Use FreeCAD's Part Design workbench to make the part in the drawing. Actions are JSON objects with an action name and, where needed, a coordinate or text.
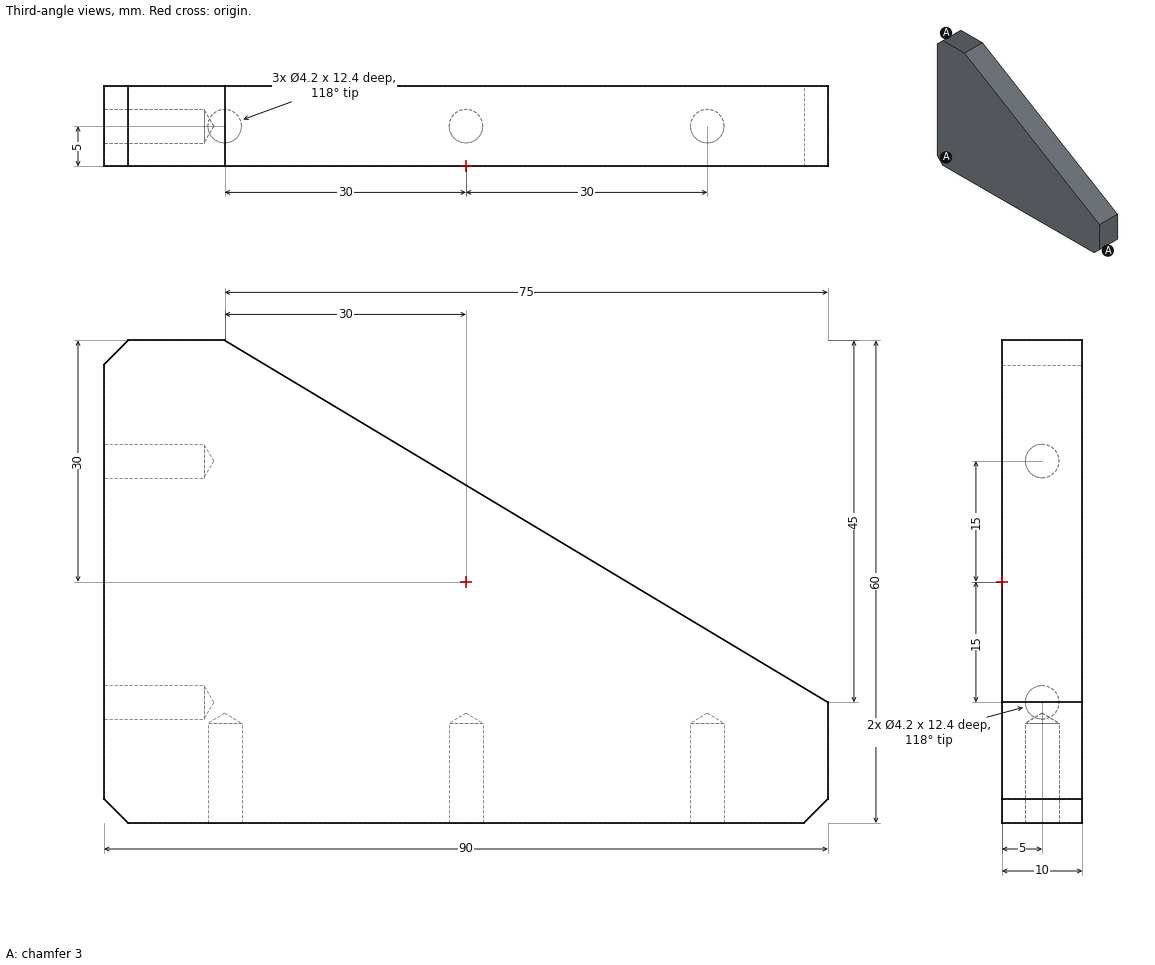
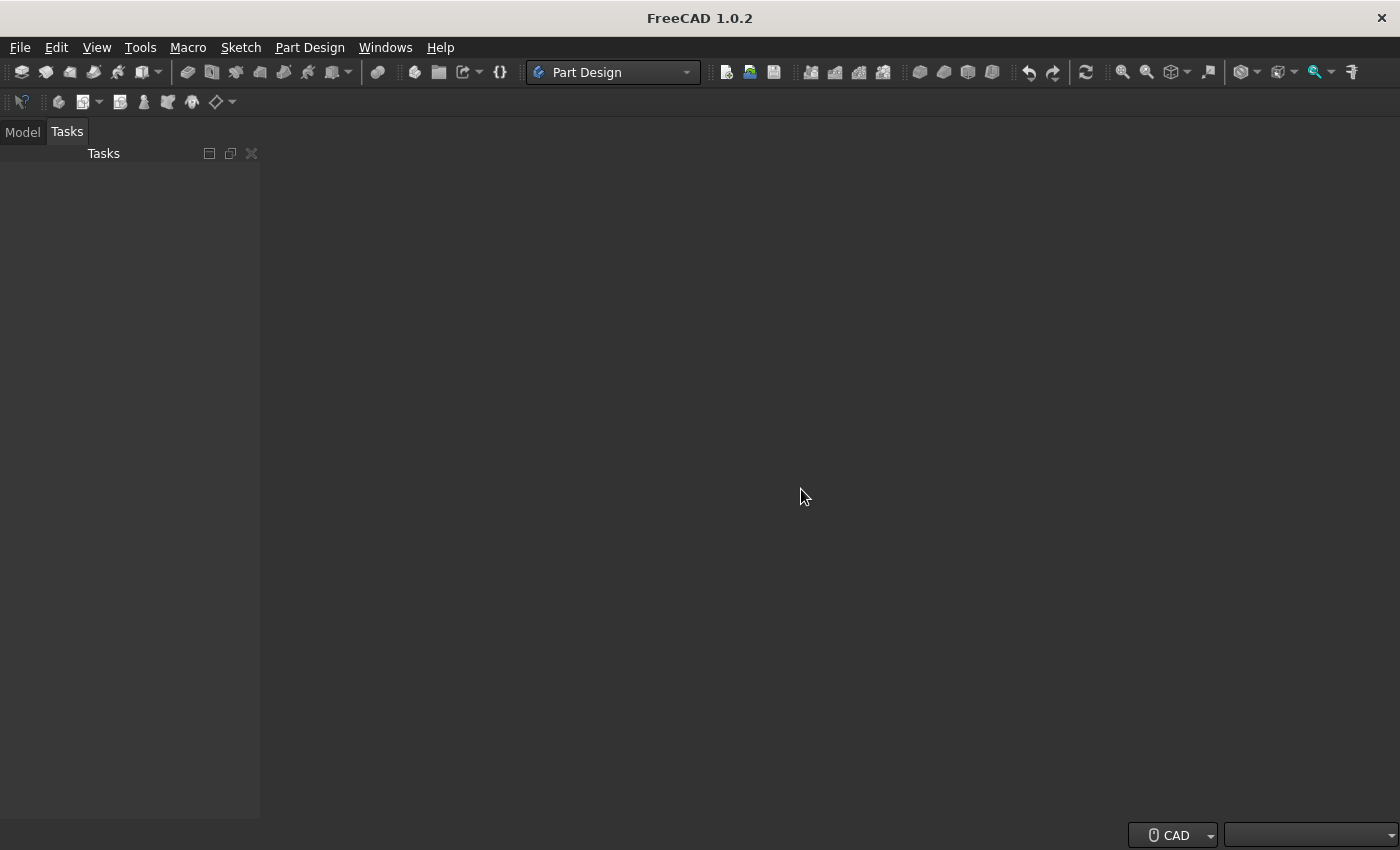
{"action": "key", "text": "ctrl+n"}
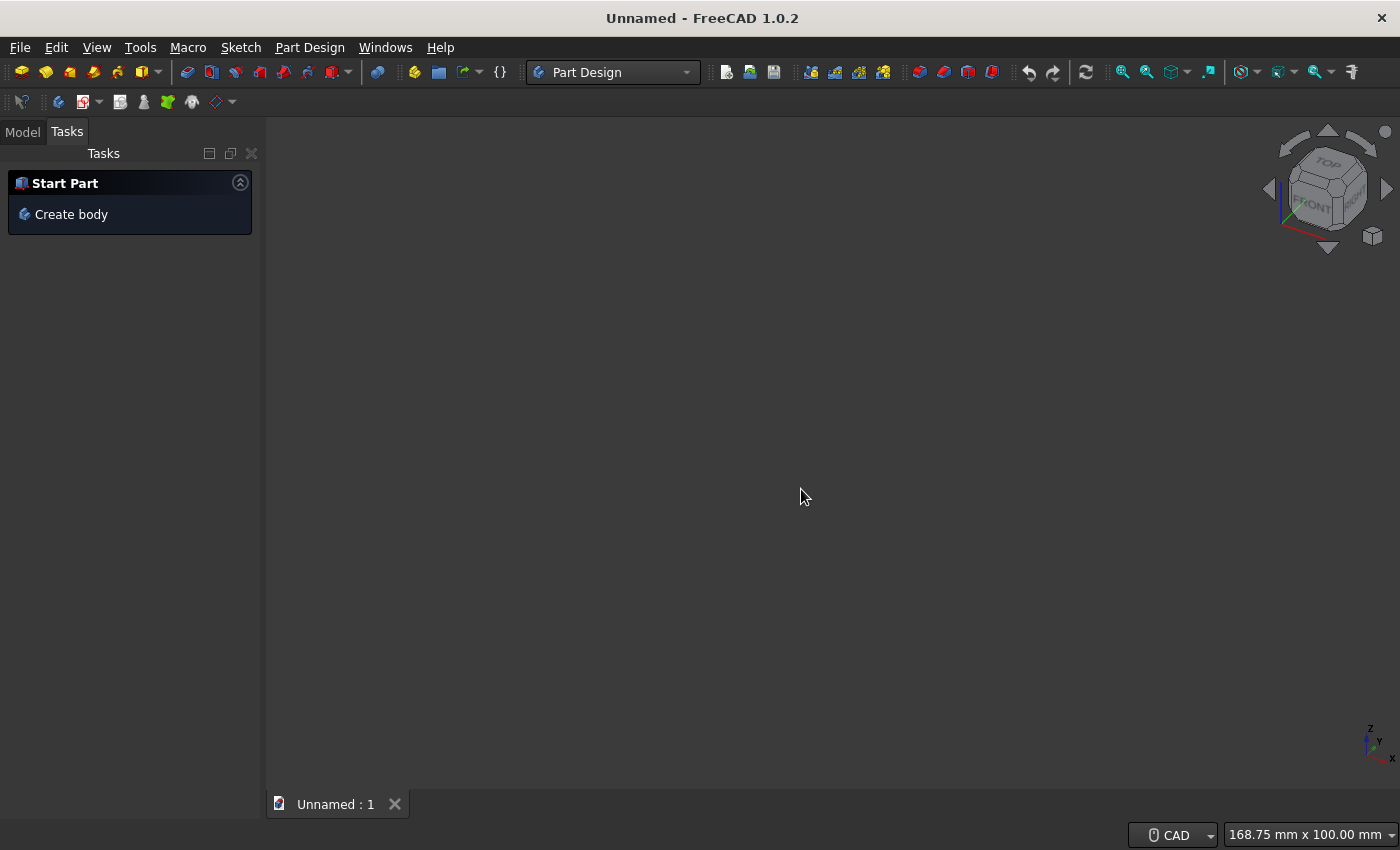
{"action": "left_click", "coordinate": [84, 102]}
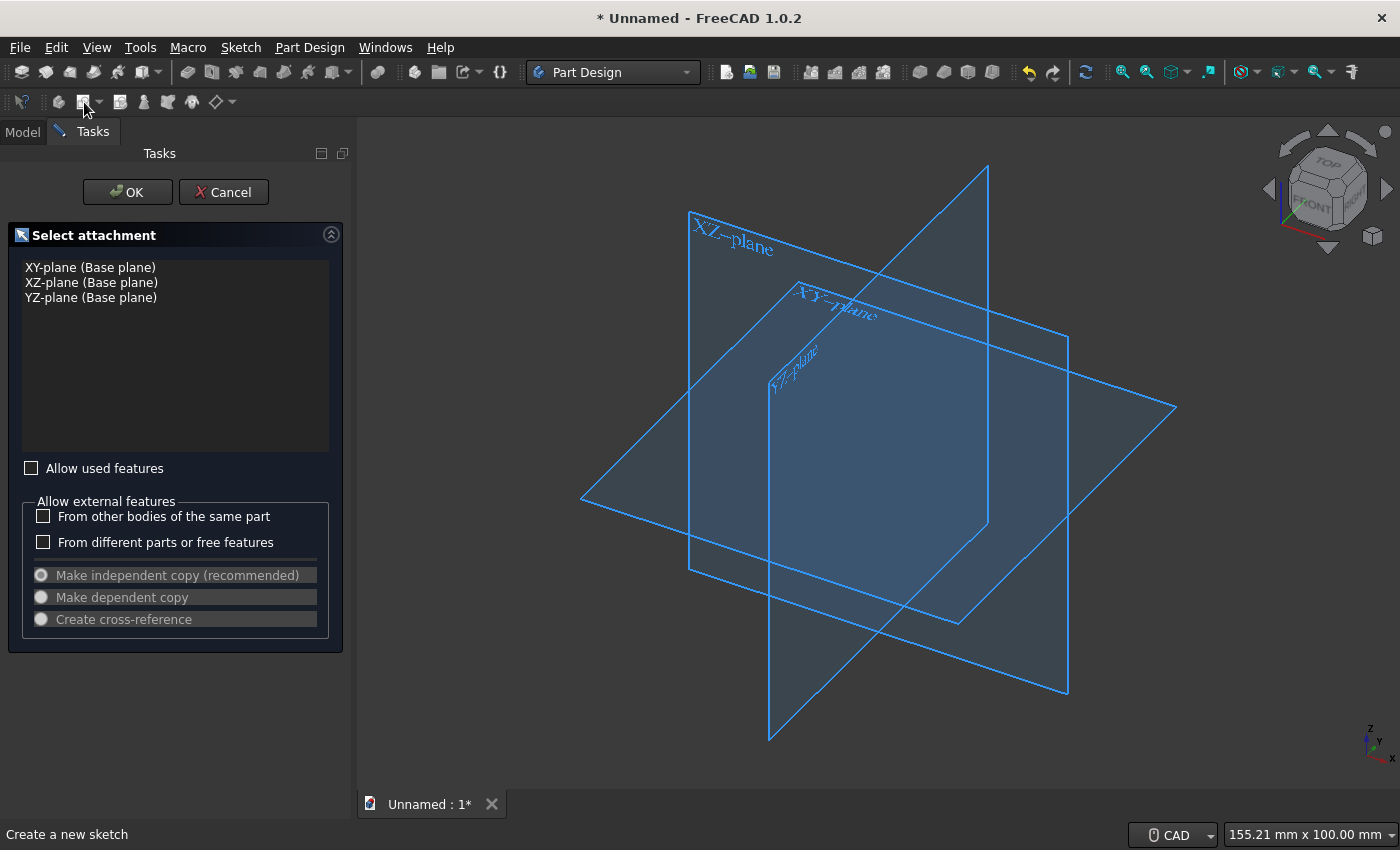
{"action": "left_click", "coordinate": [82, 282]}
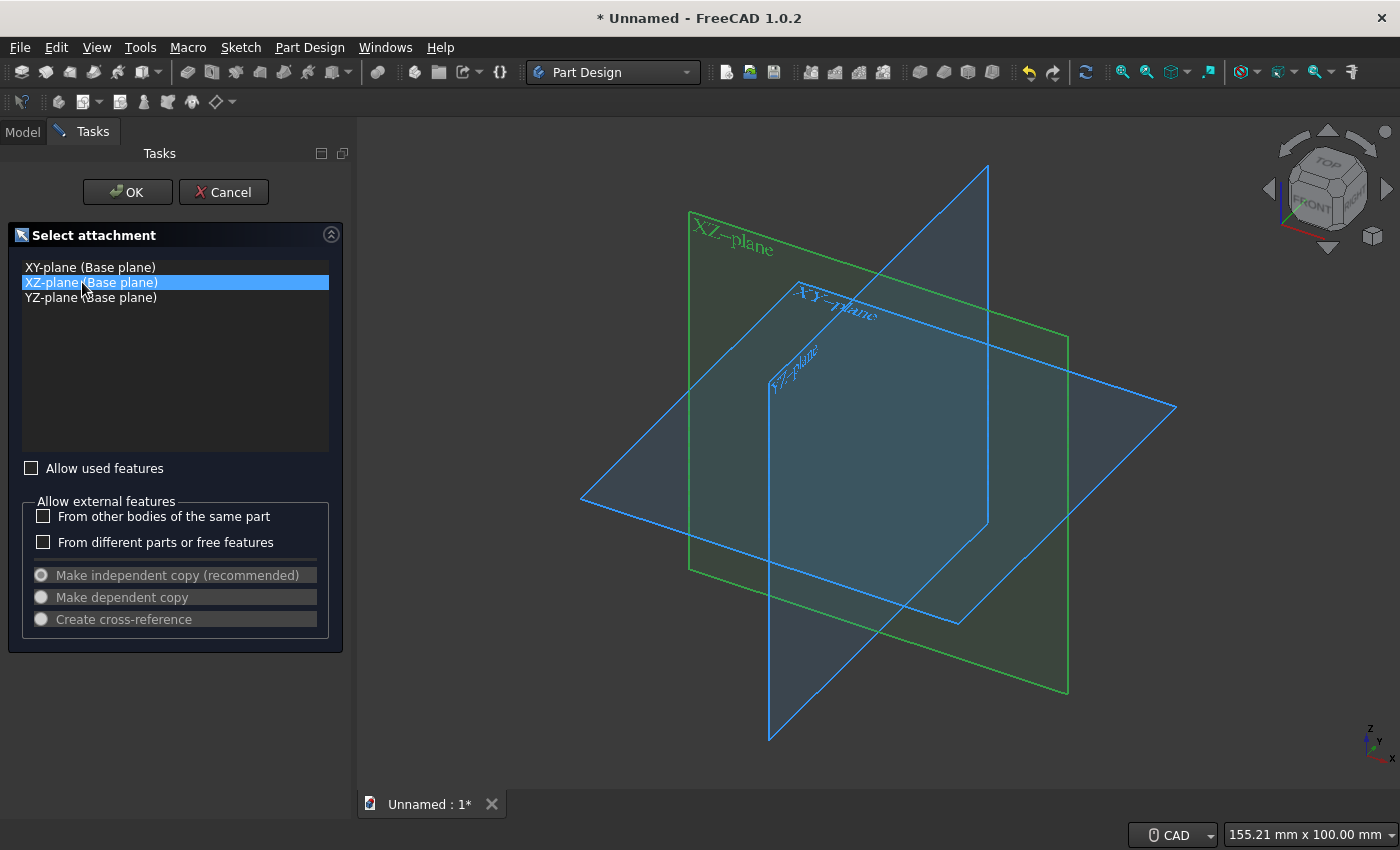
{"action": "left_click", "coordinate": [128, 192]}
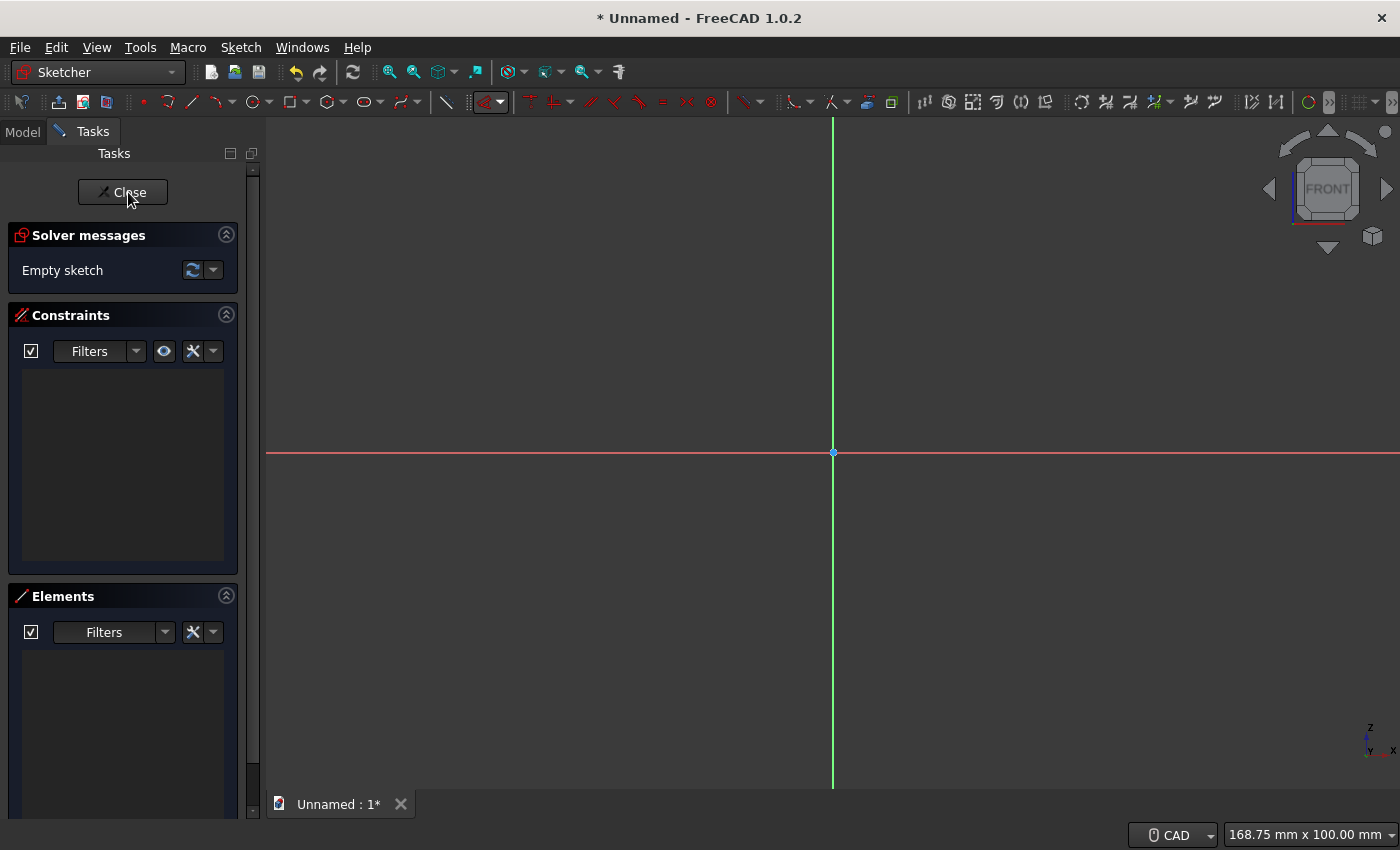
{"action": "key", "text": "g v"}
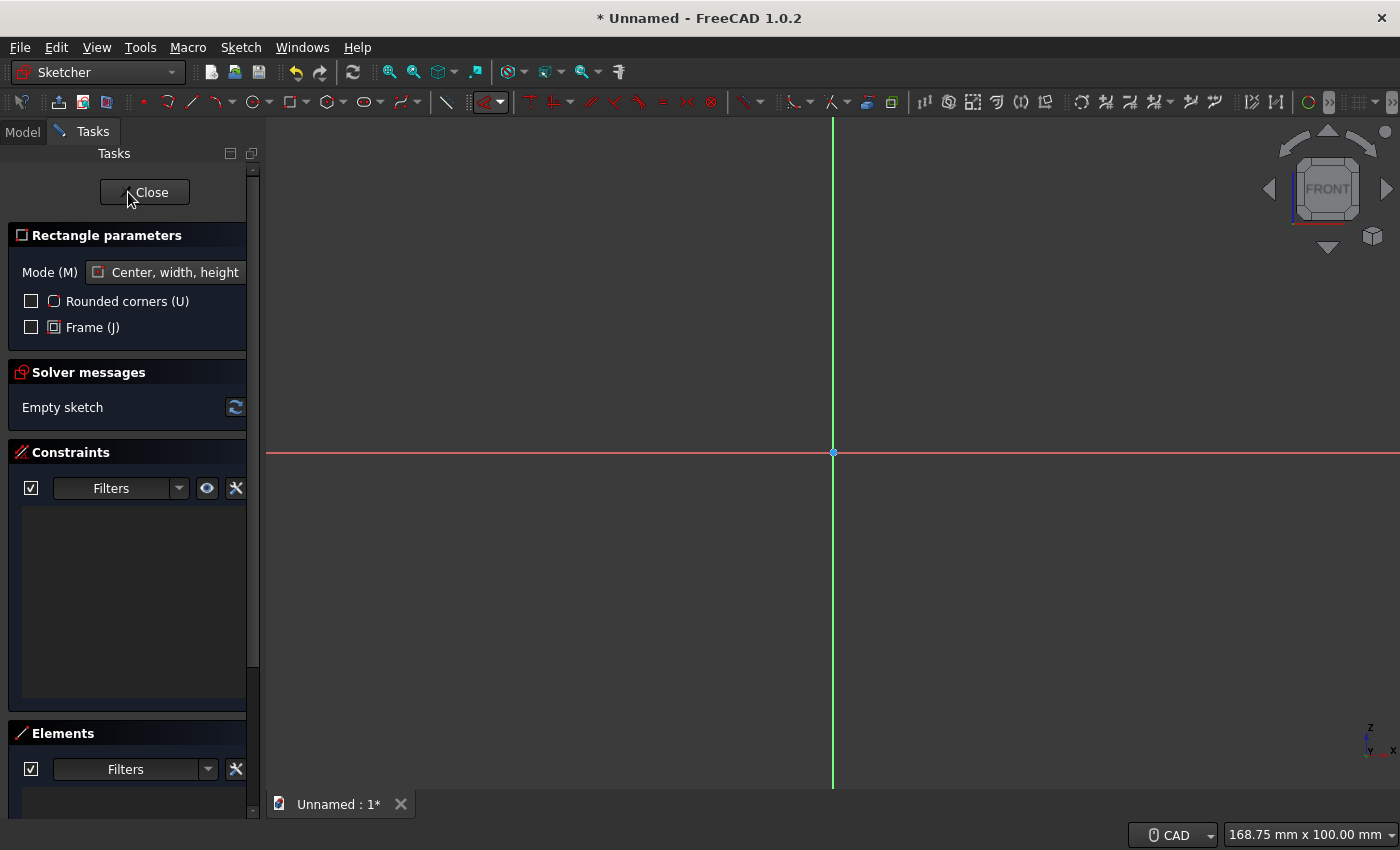
{"action": "left_click", "coordinate": [833, 453]}
{"action": "mouse_move", "coordinate": [1135, 251]}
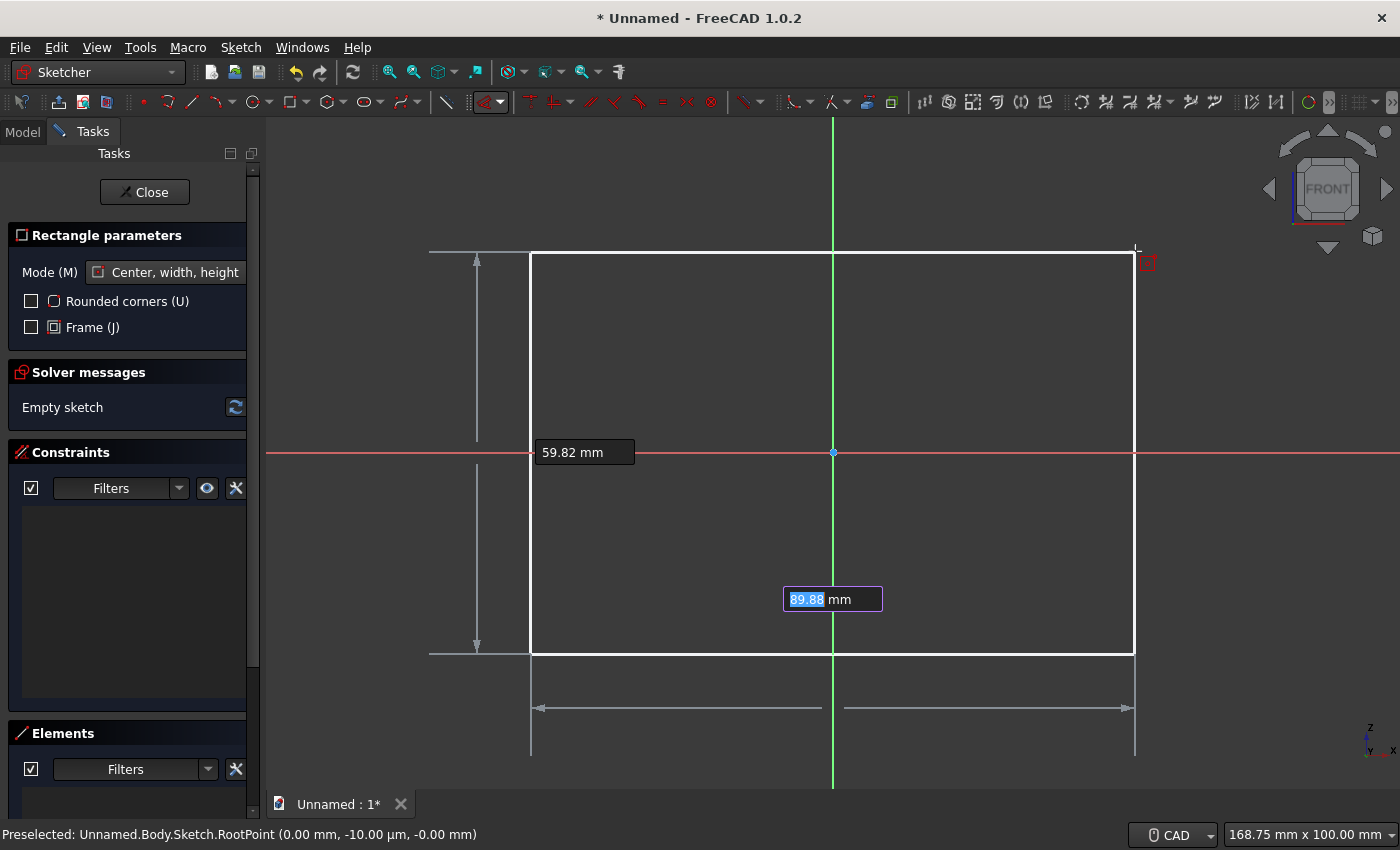
{"action": "type", "text": "90"}
{"action": "key", "text": "Tab"}
{"action": "type", "text": "60"}
{"action": "key", "text": "Return"}
{"action": "key", "text": "Escape"}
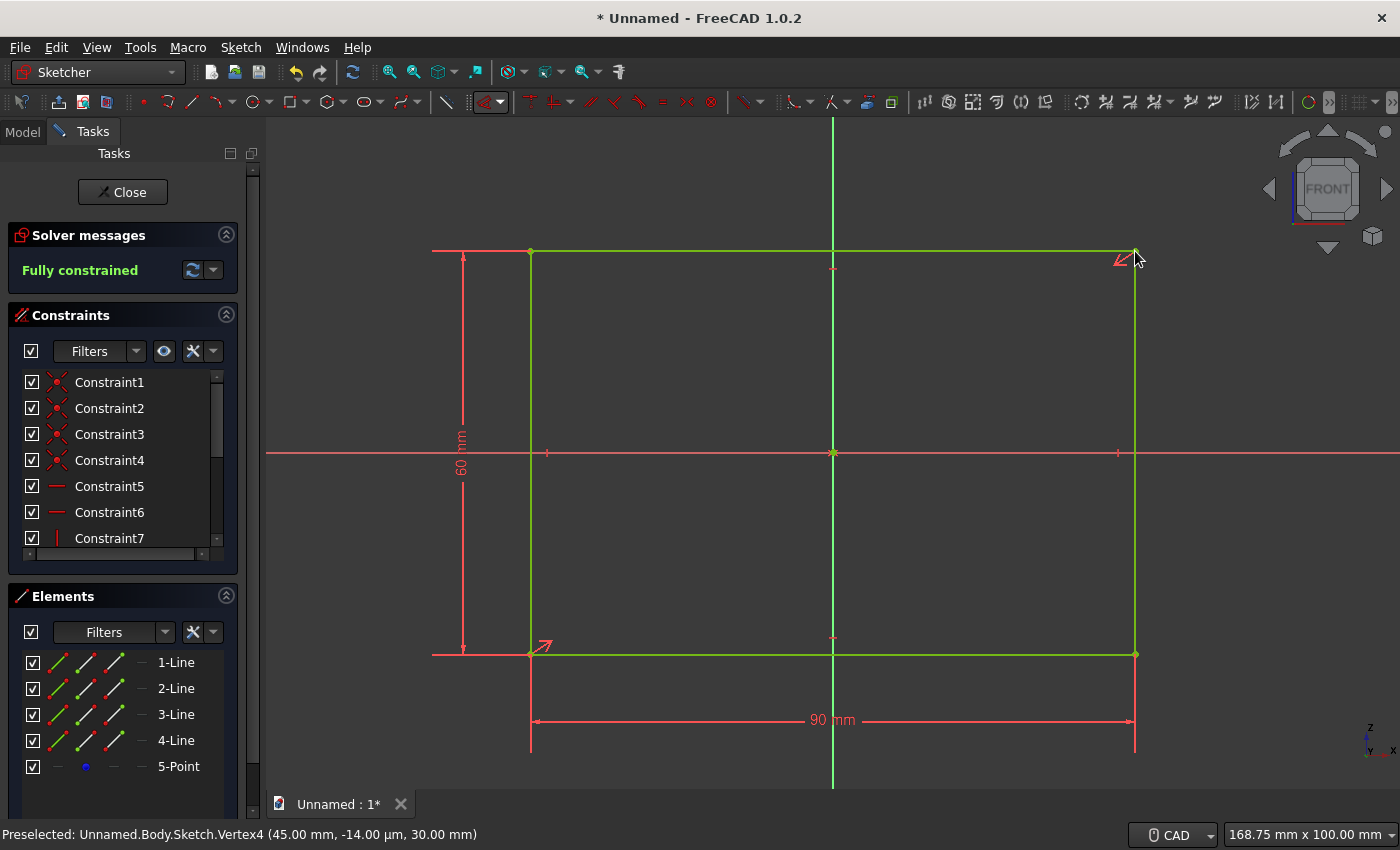
{"action": "left_click", "coordinate": [123, 192]}